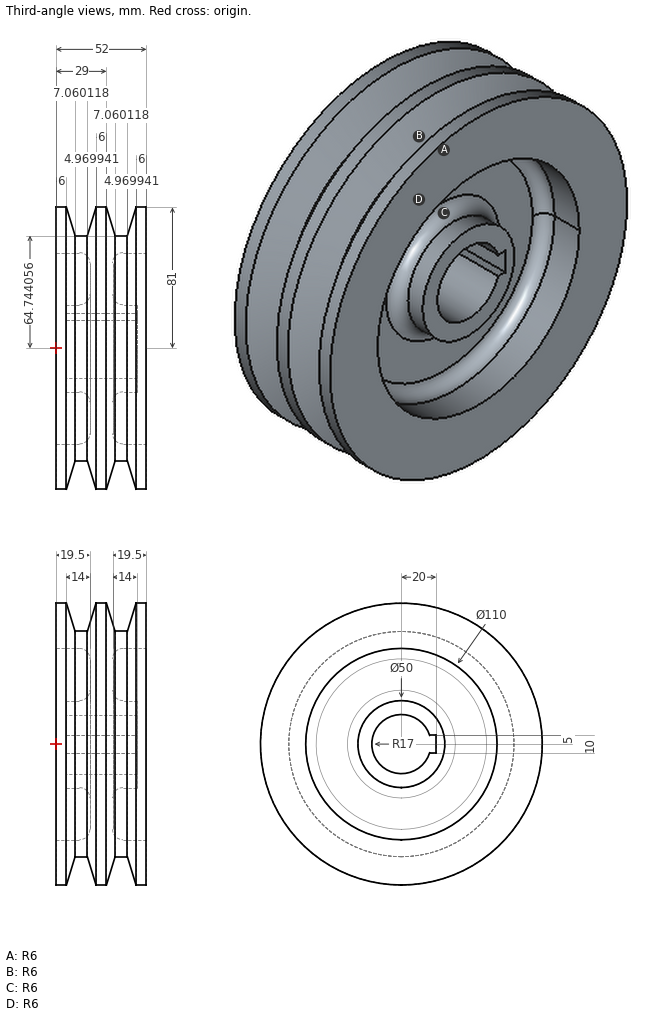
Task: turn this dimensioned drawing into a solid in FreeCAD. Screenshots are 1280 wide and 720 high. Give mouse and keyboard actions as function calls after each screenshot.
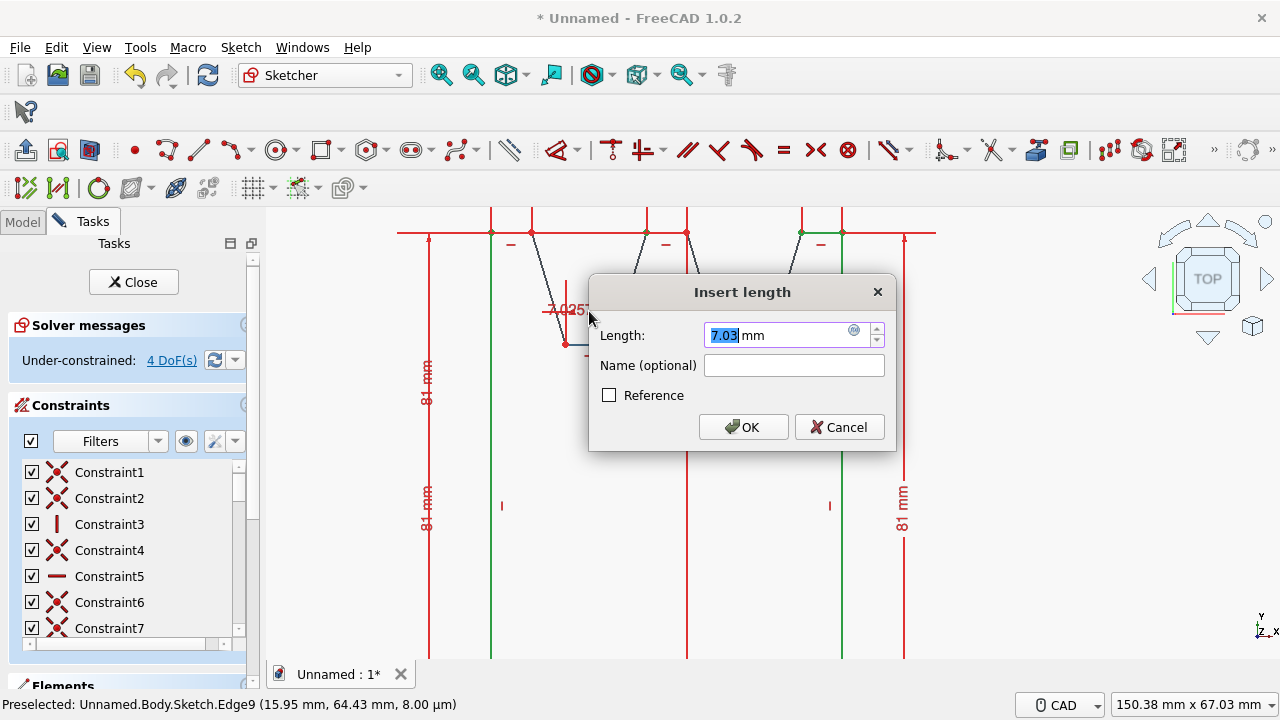
text(7.060118)
key(Return)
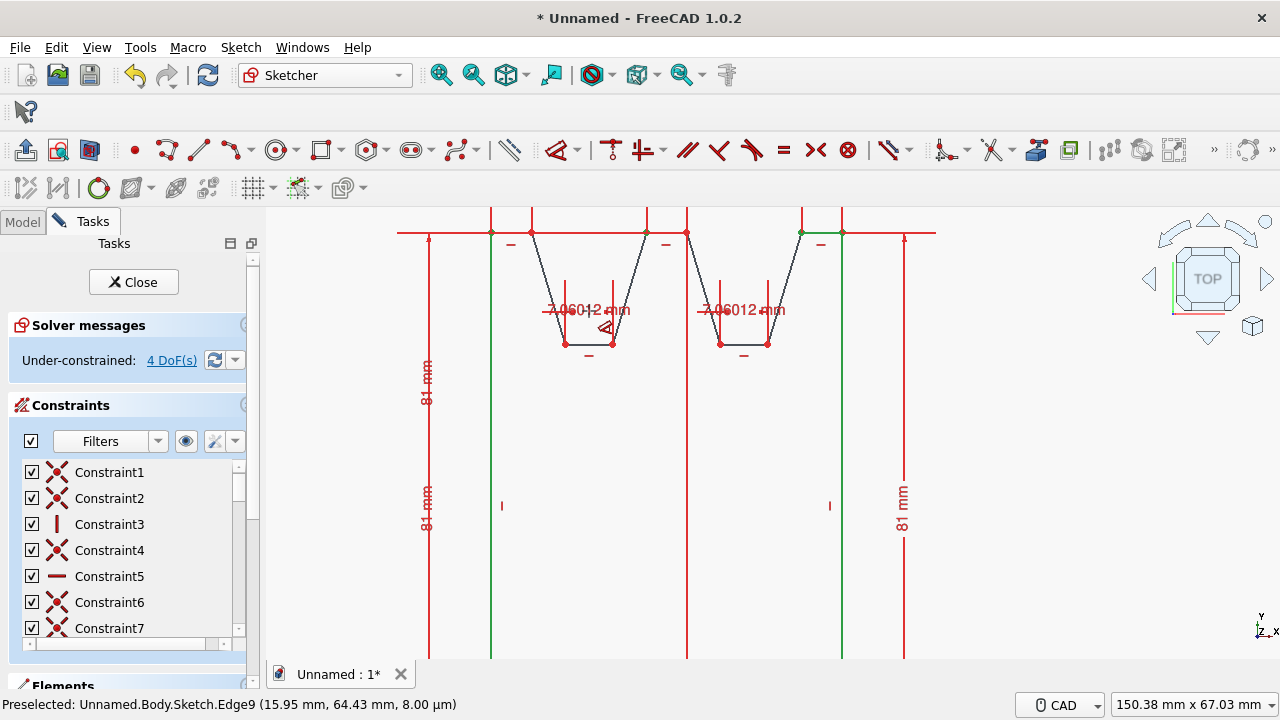
click(791, 266)
click(785, 379)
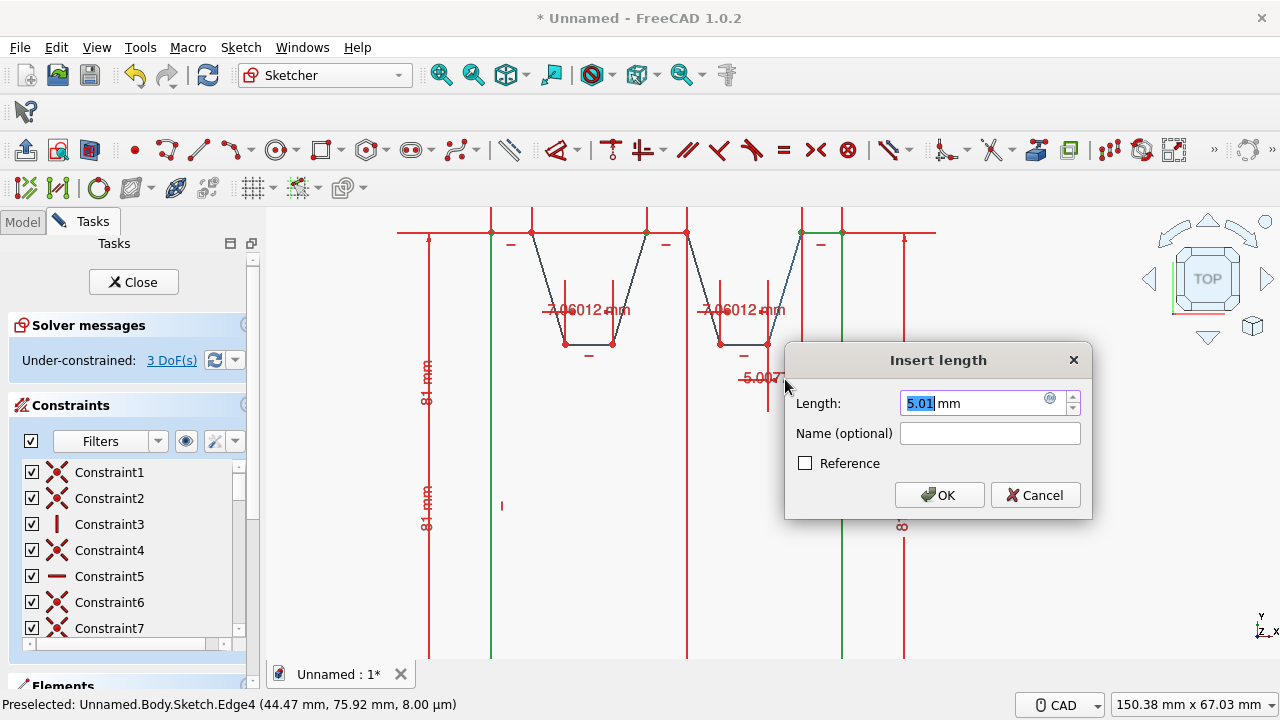
text(4.969941)
key(Return)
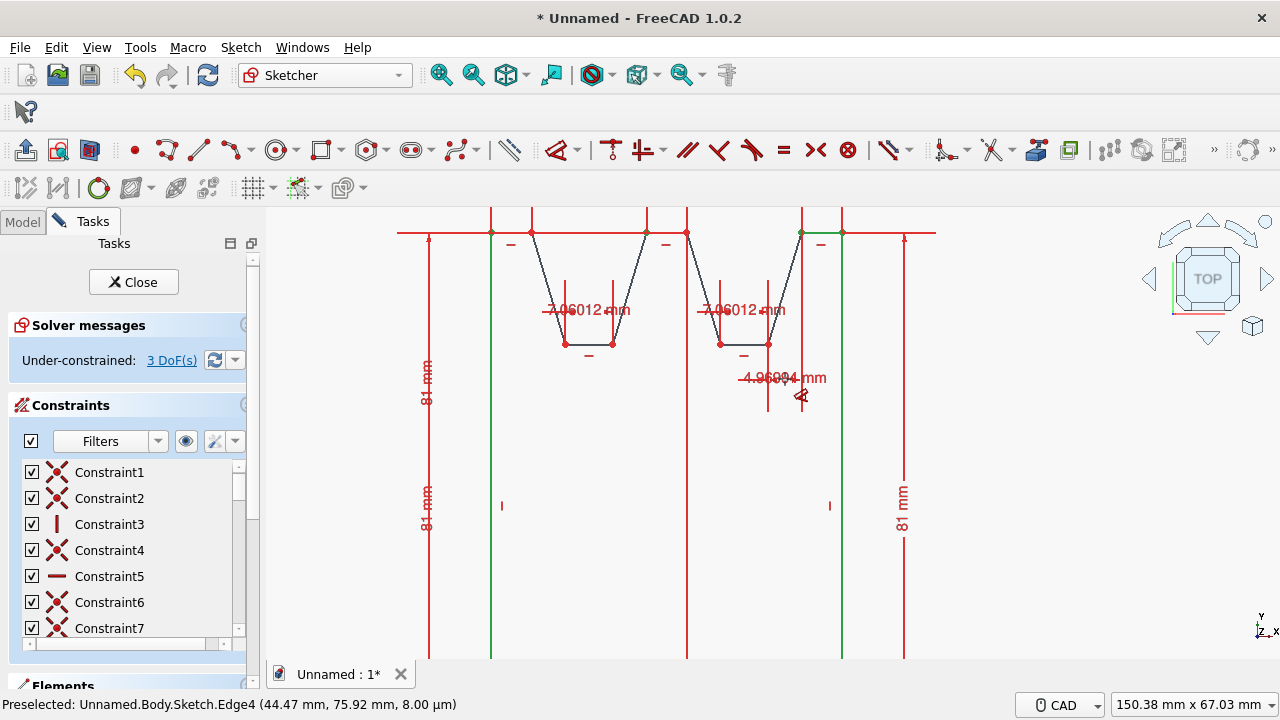
click(636, 266)
click(630, 379)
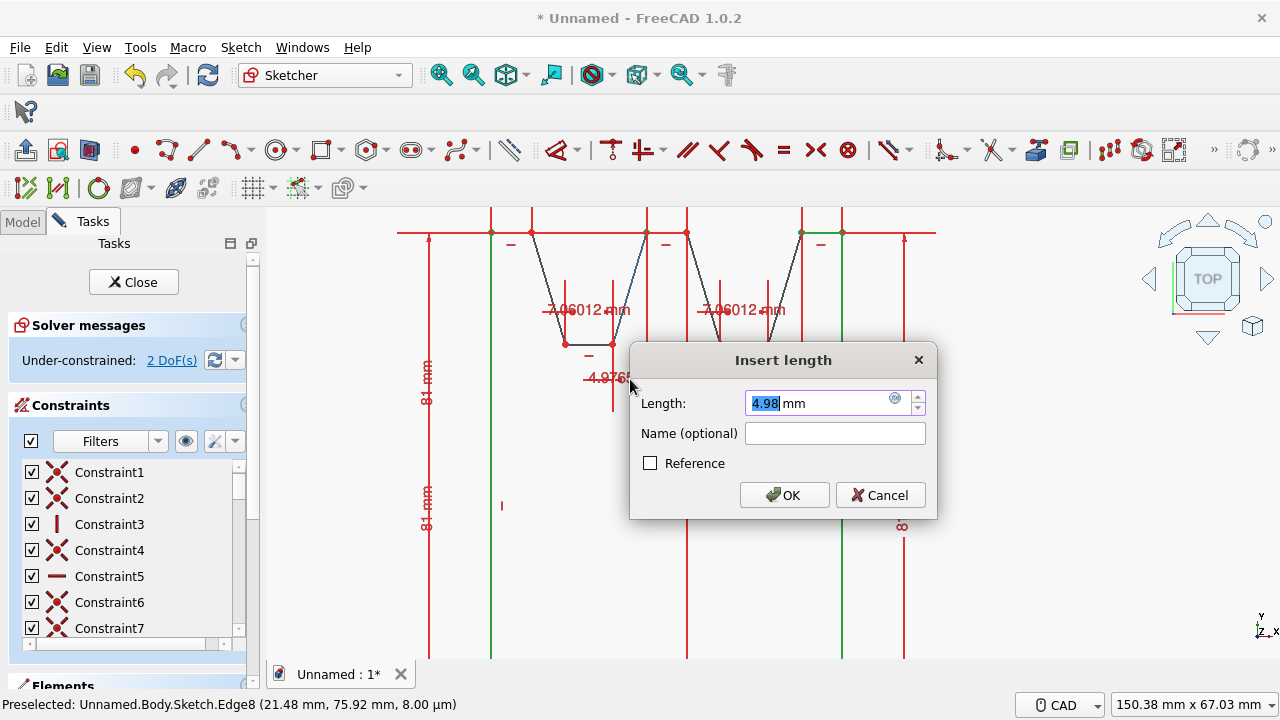
text(4.969941)
key(Return)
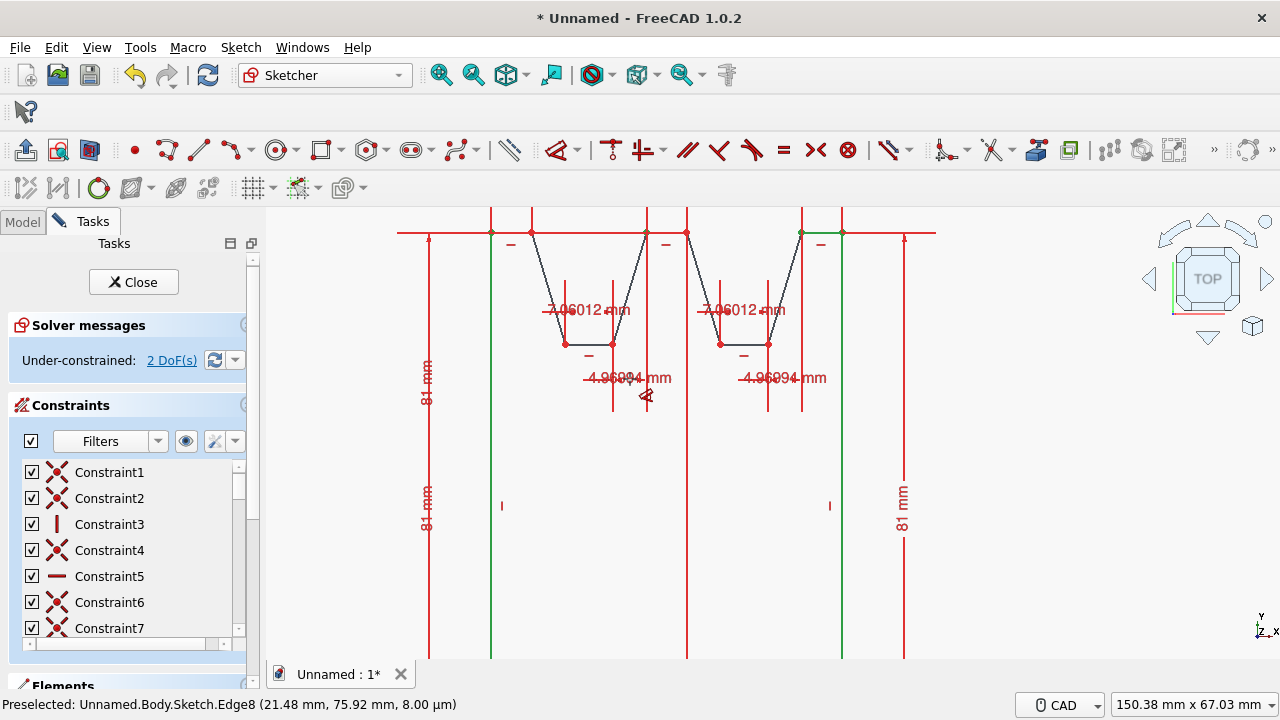
click(768, 345)
click(457, 422)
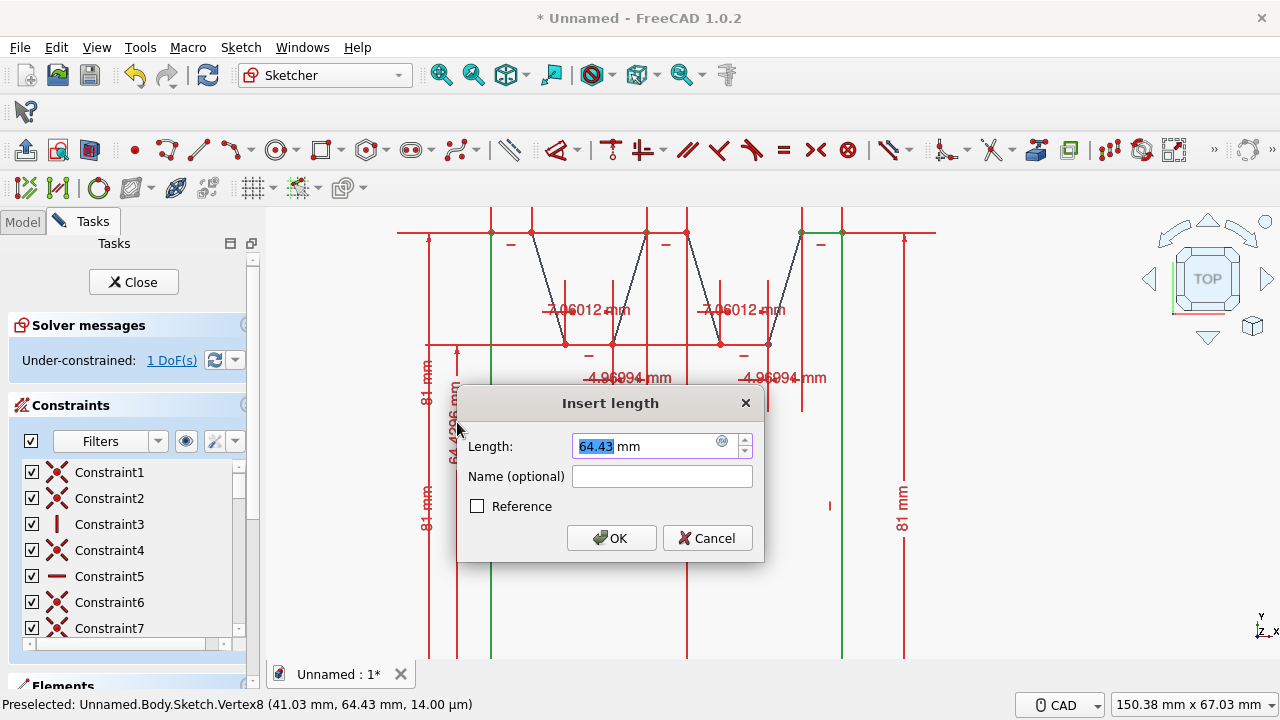
text(64.744056)
key(Return)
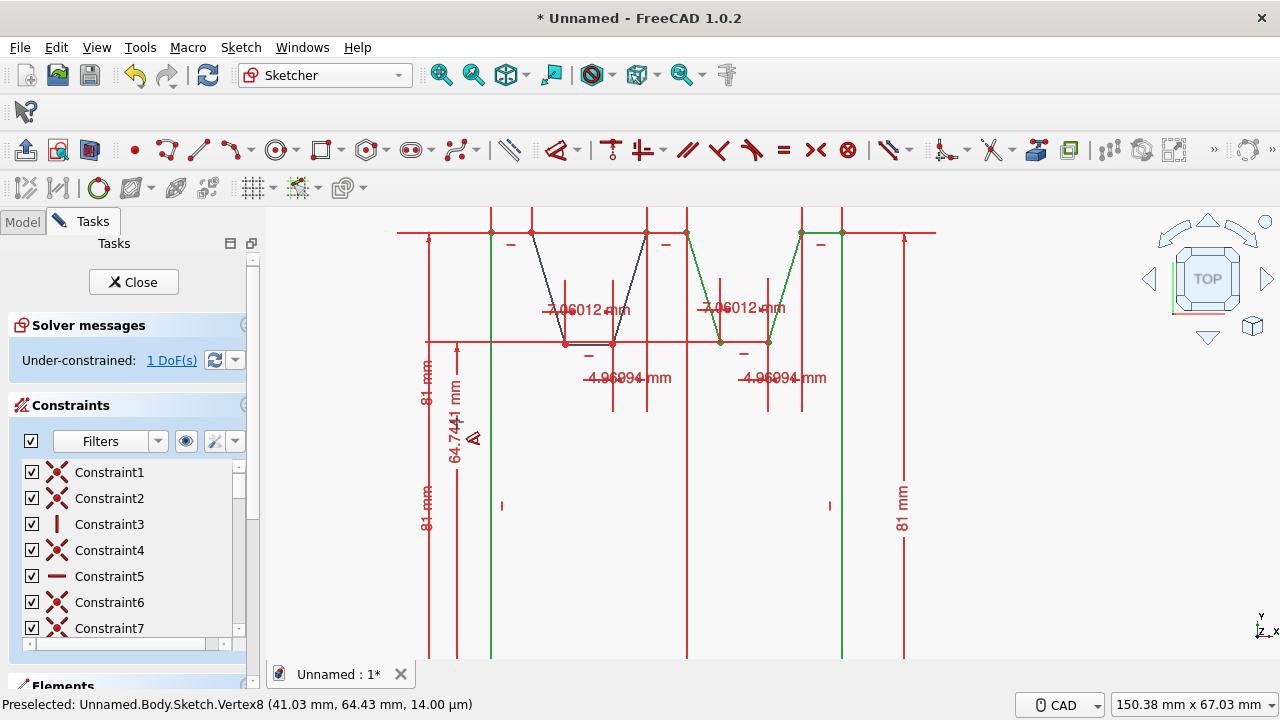
click(613, 345)
click(457, 554)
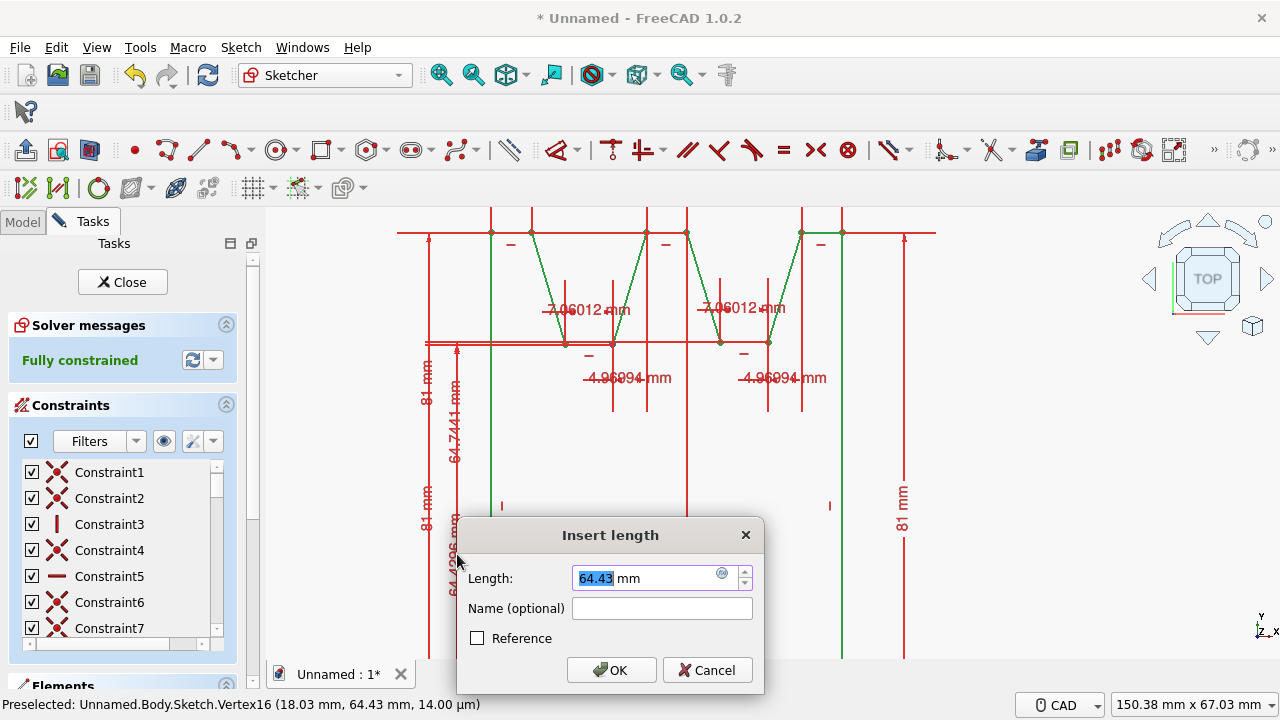
text(64.744056)
key(Return)
key(Escape)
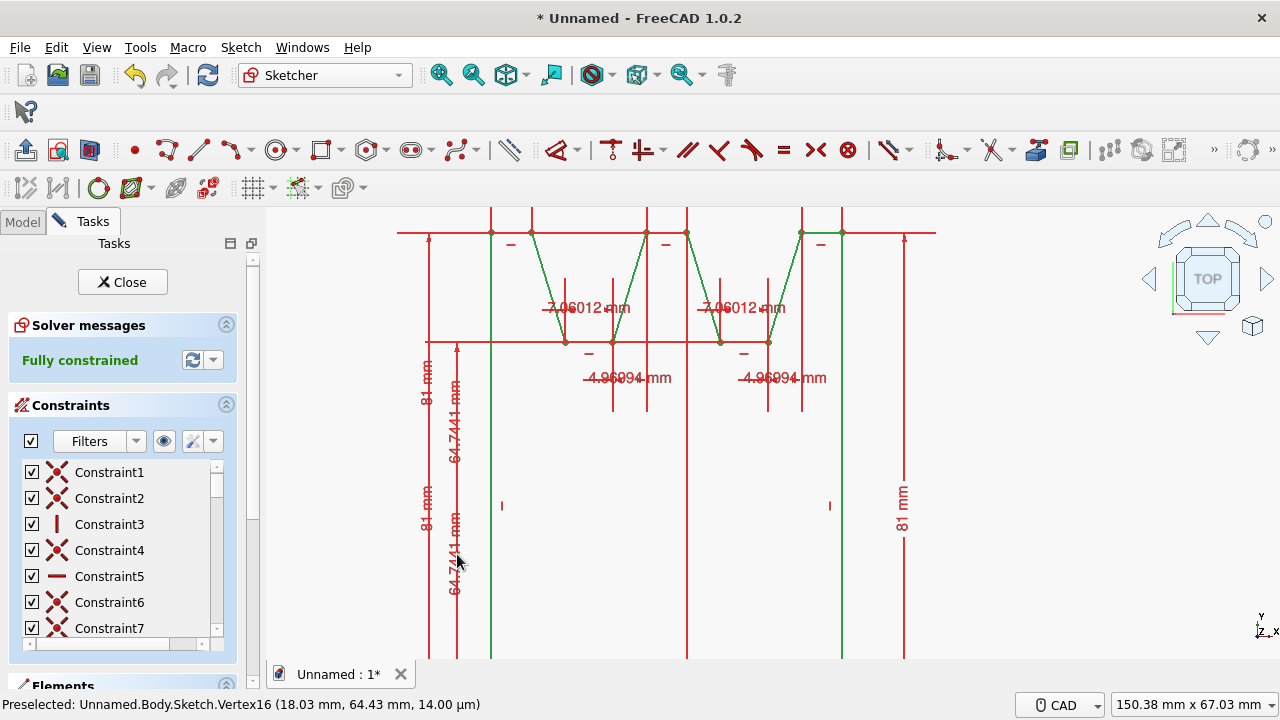
click(123, 282)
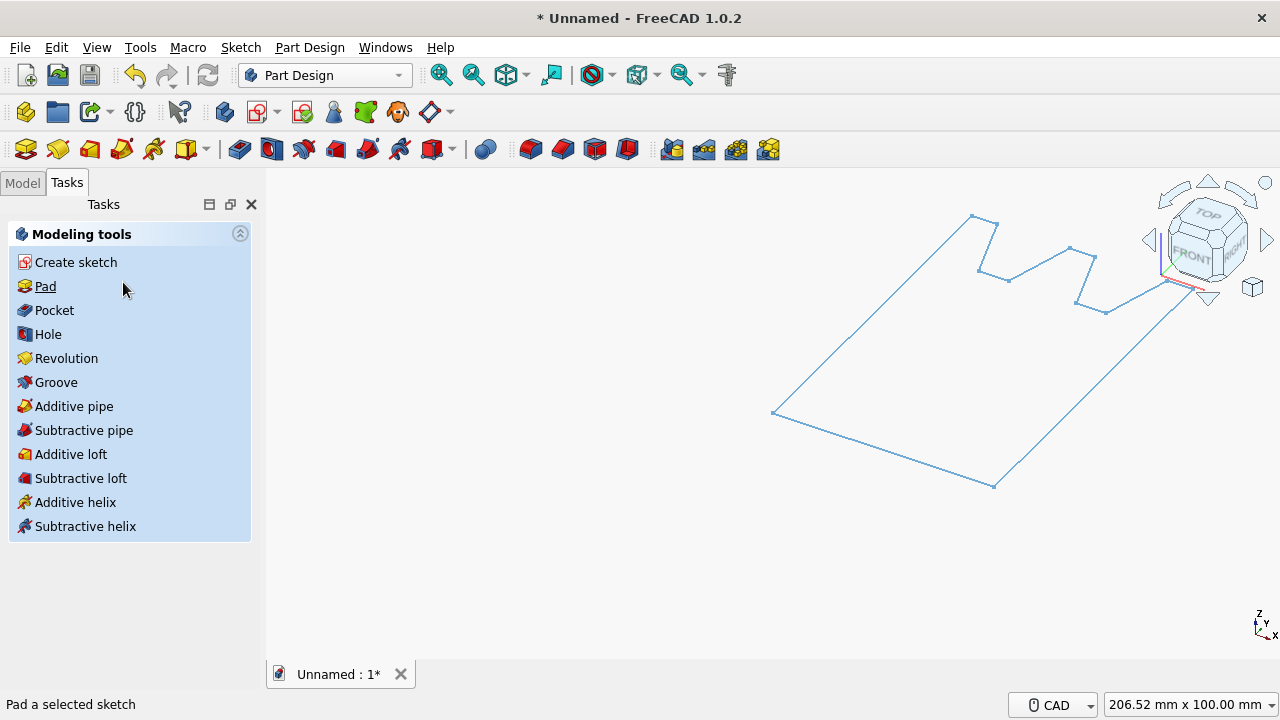
click(58, 150)